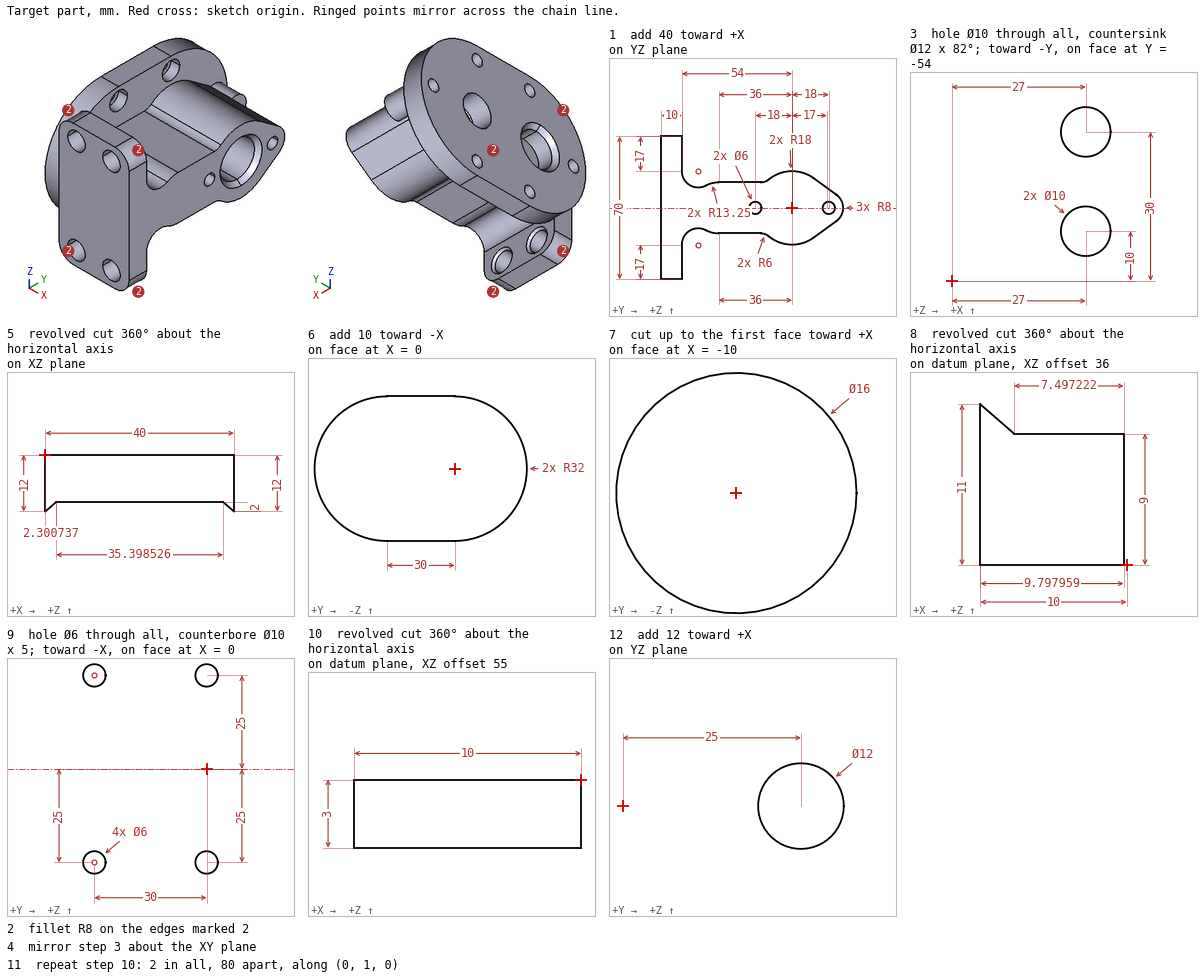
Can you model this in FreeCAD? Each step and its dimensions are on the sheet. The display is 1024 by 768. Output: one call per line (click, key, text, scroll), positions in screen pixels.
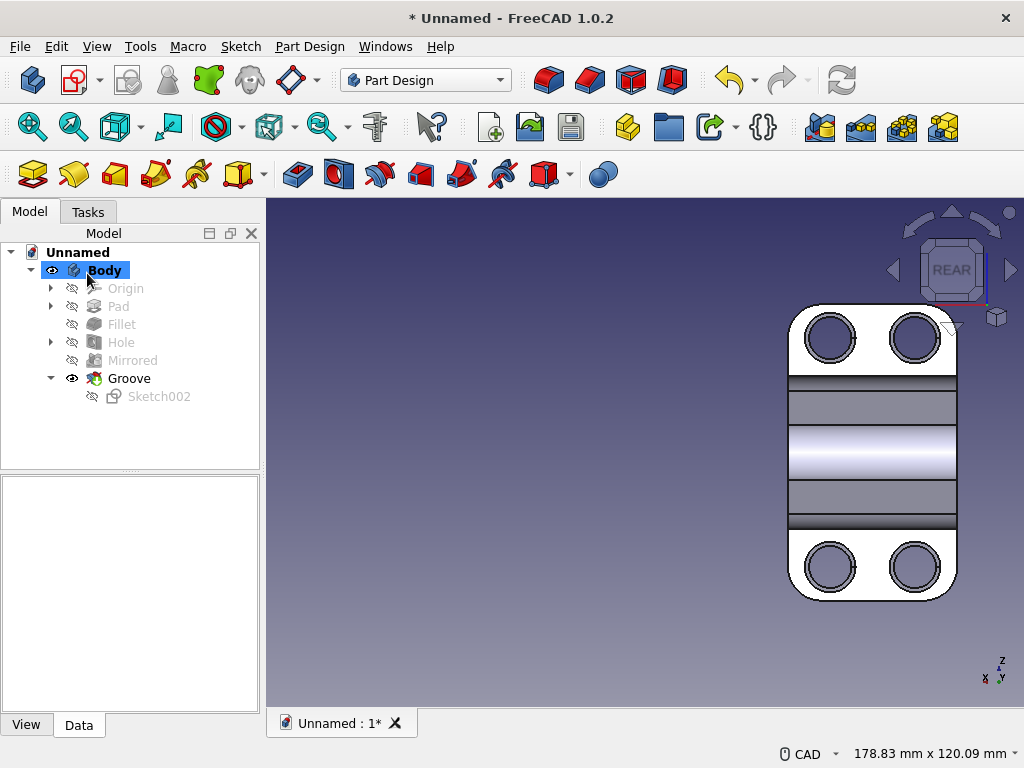
key(6)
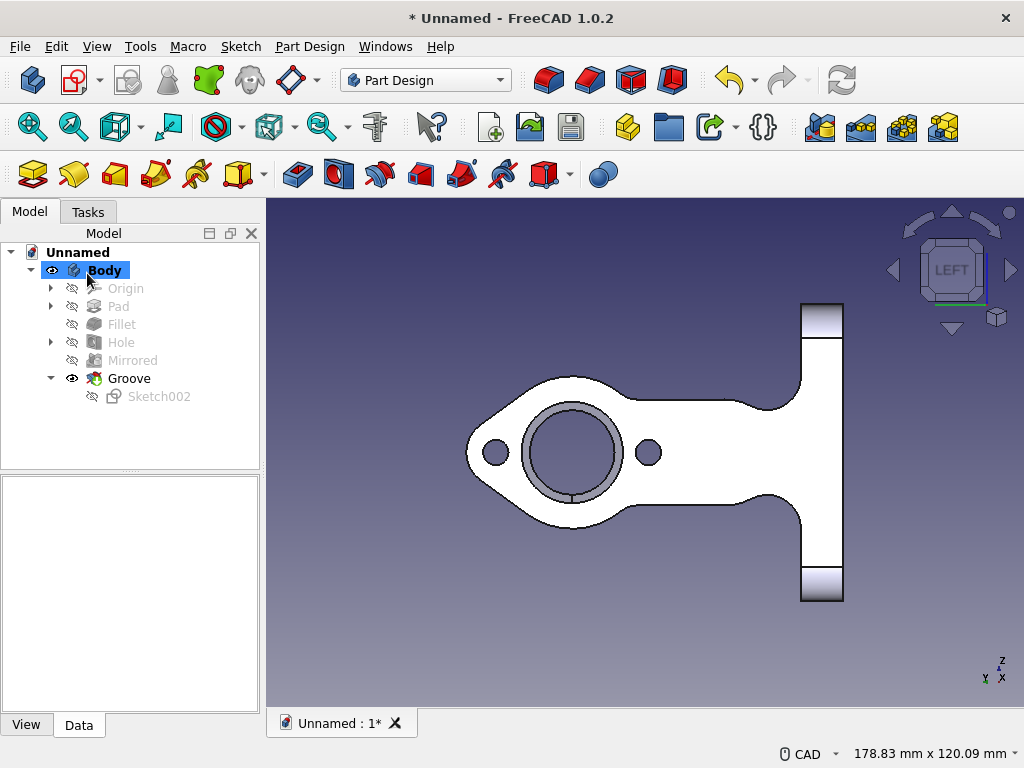
click(709, 451)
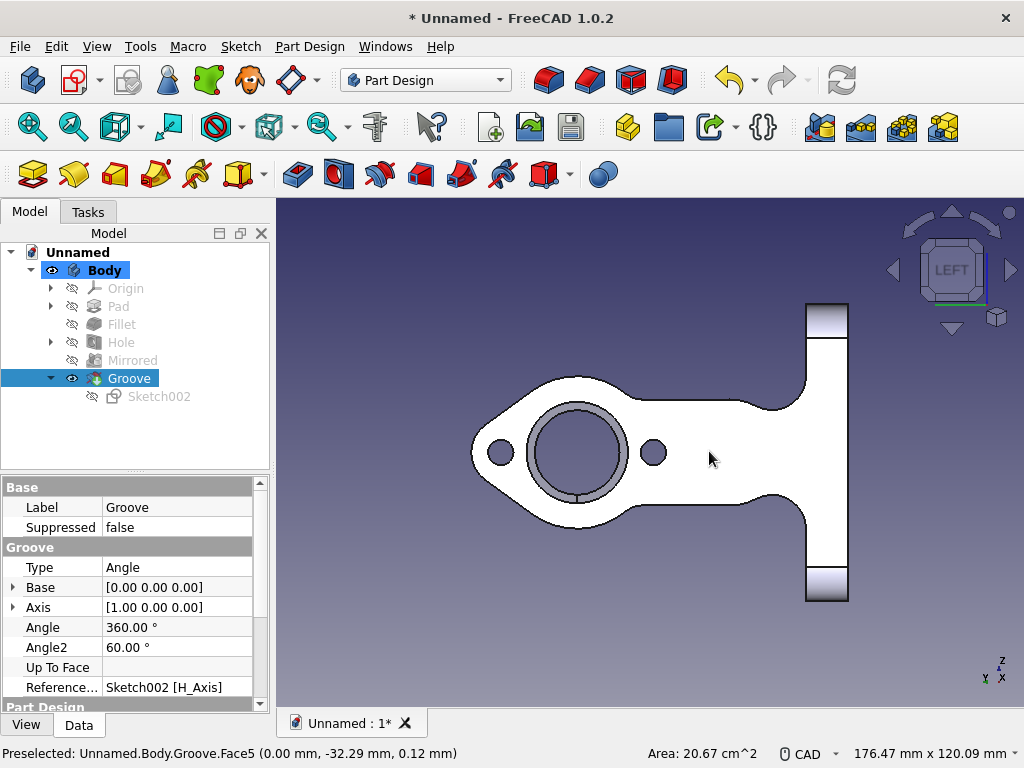
click(74, 80)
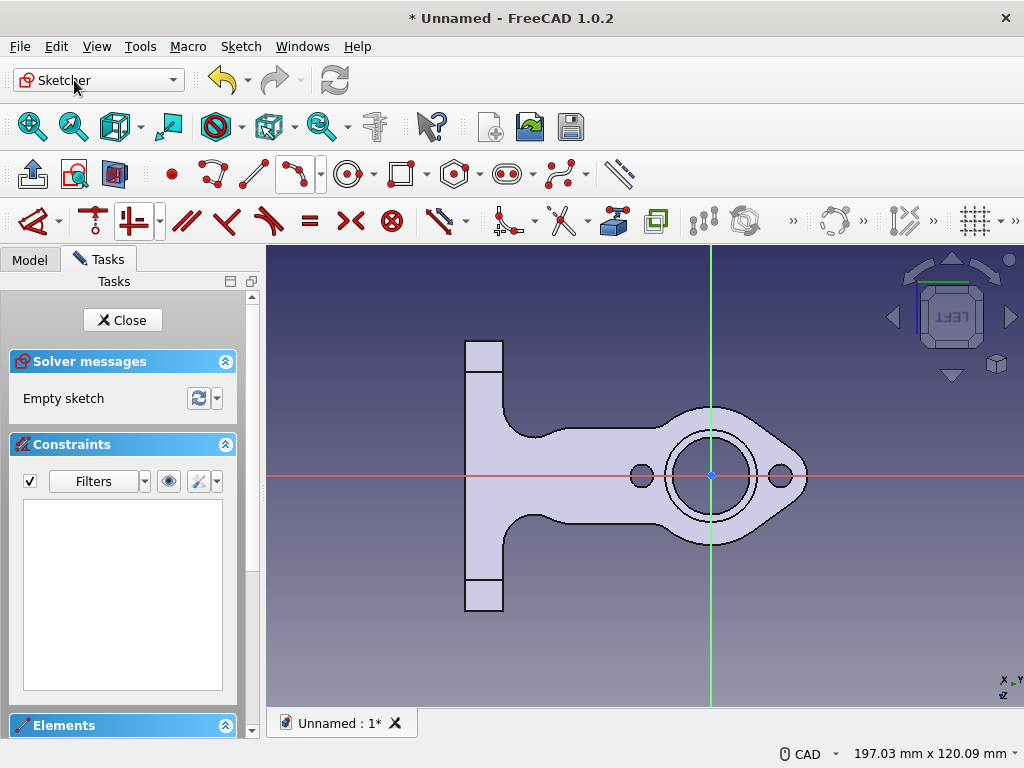
scroll(294, 476, down, 1)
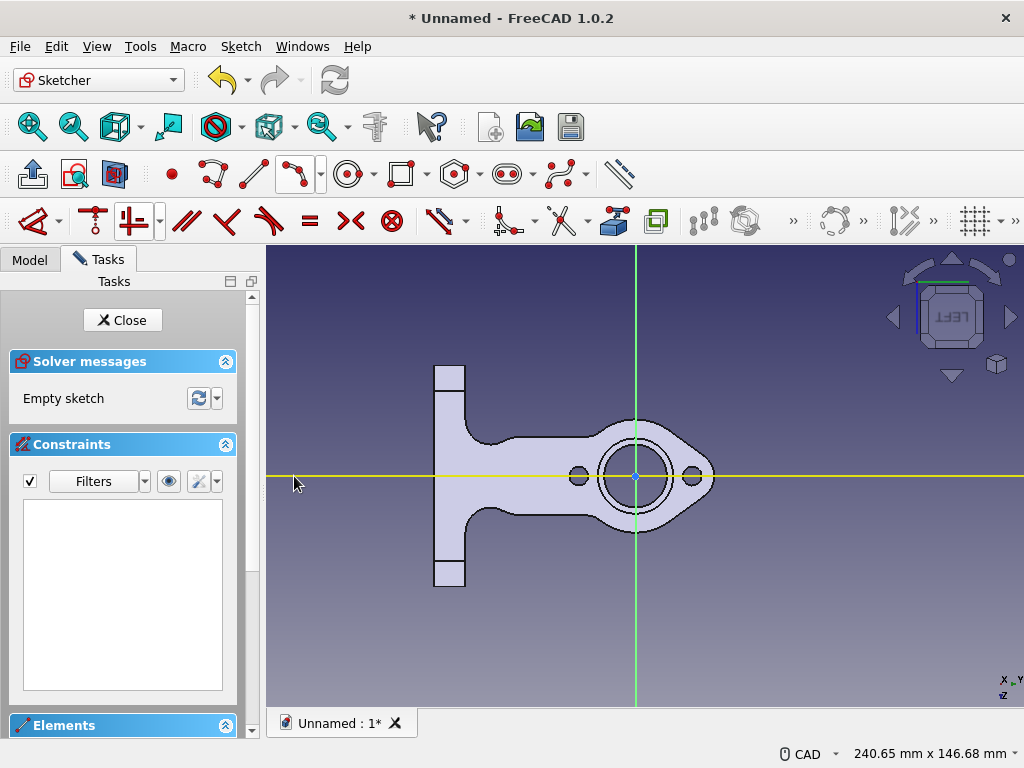
click(506, 174)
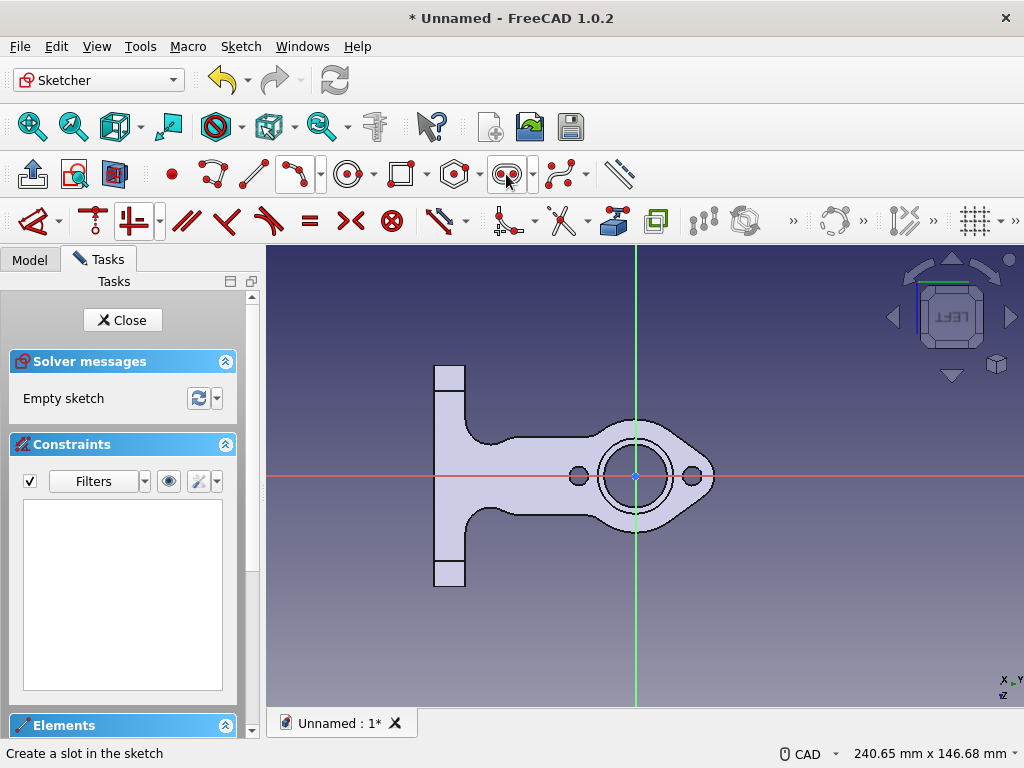
click(636, 476)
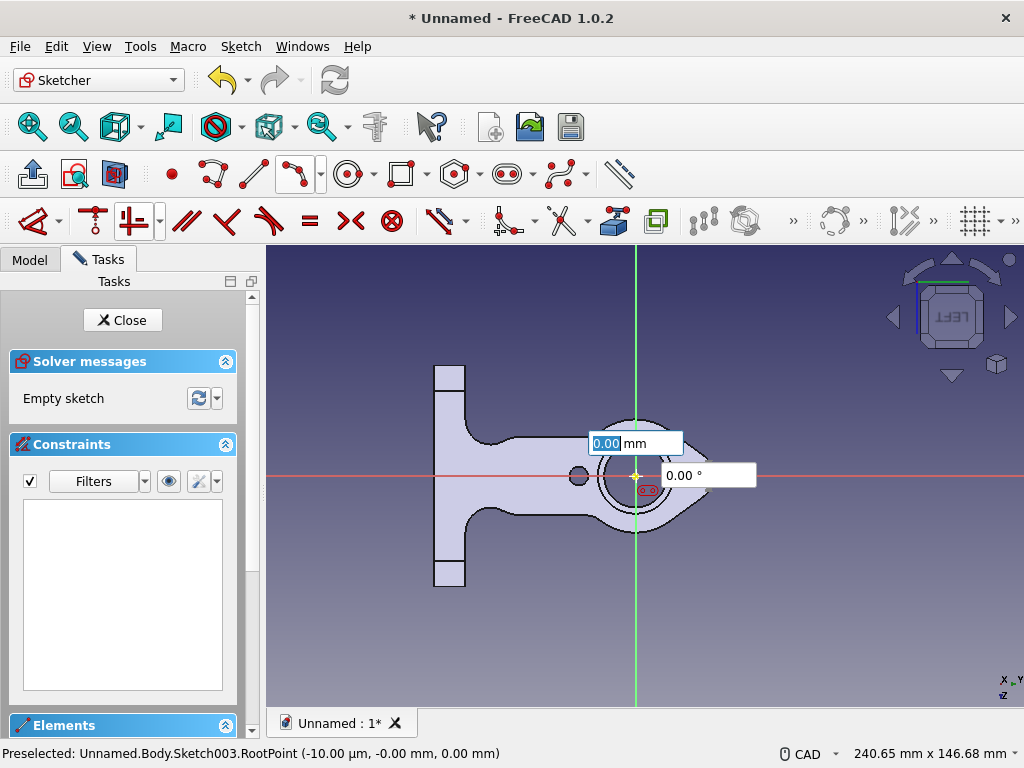
click(541, 467)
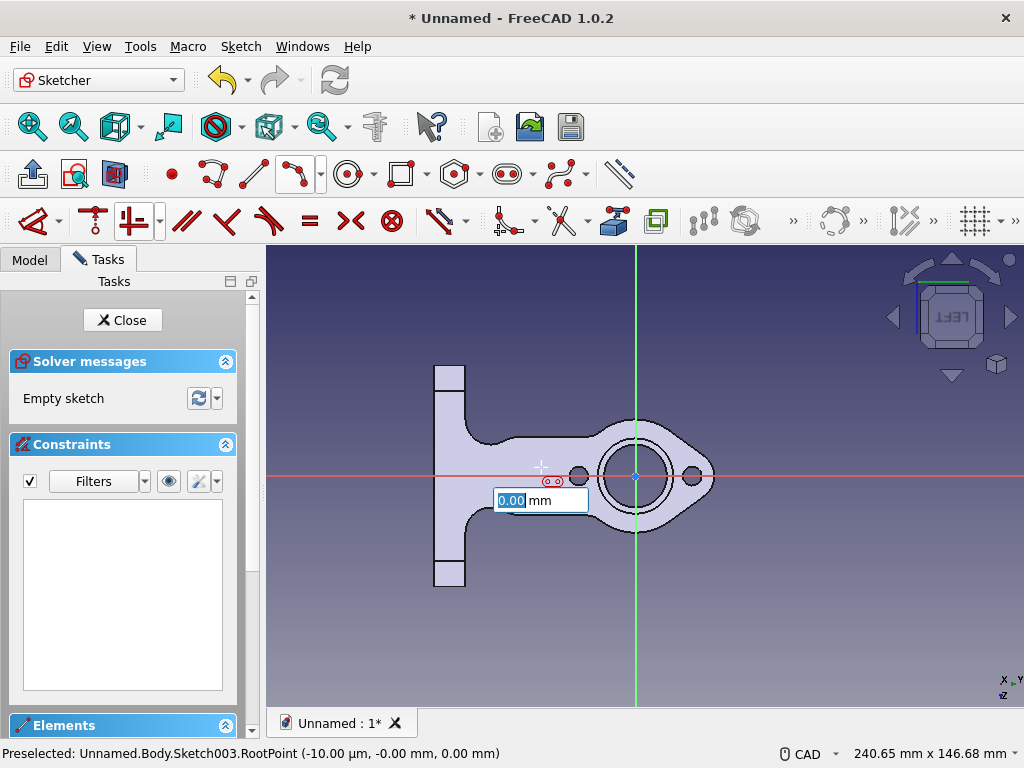
click(588, 577)
key(Escape)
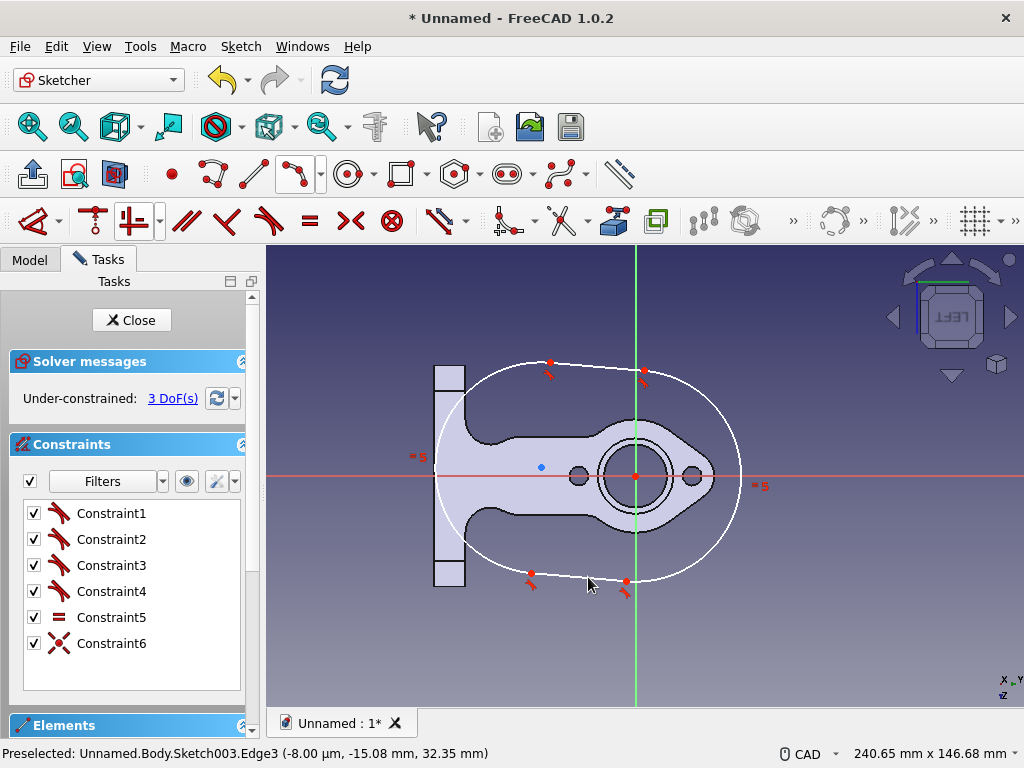
click(598, 579)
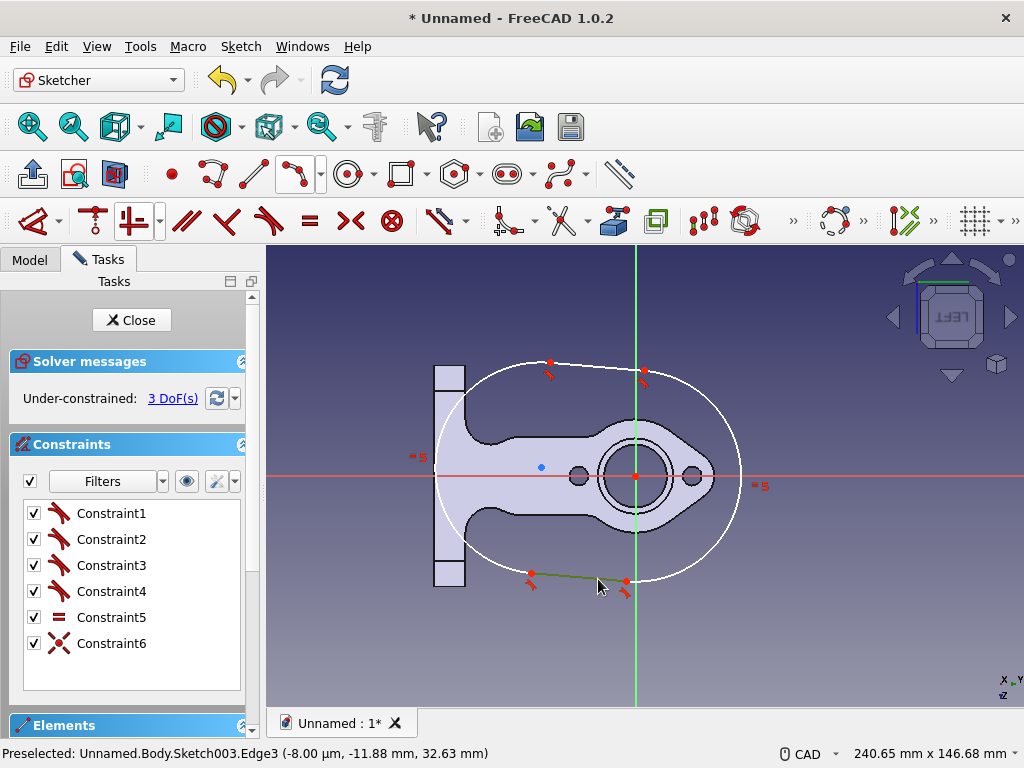
click(160, 222)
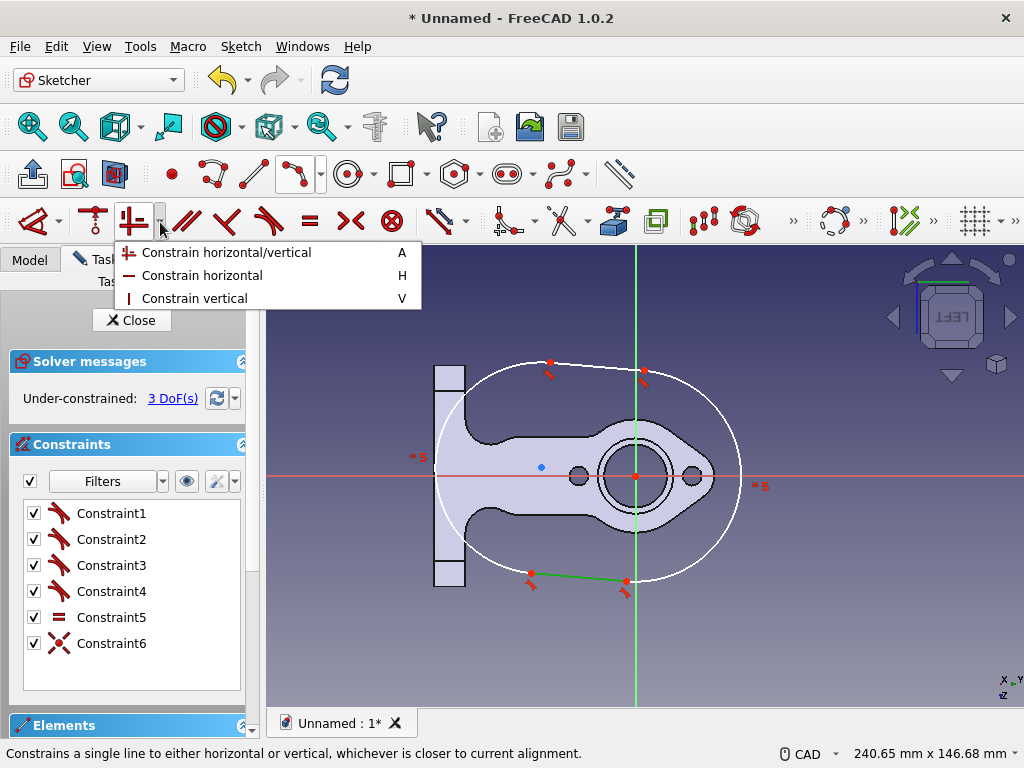
click(268, 276)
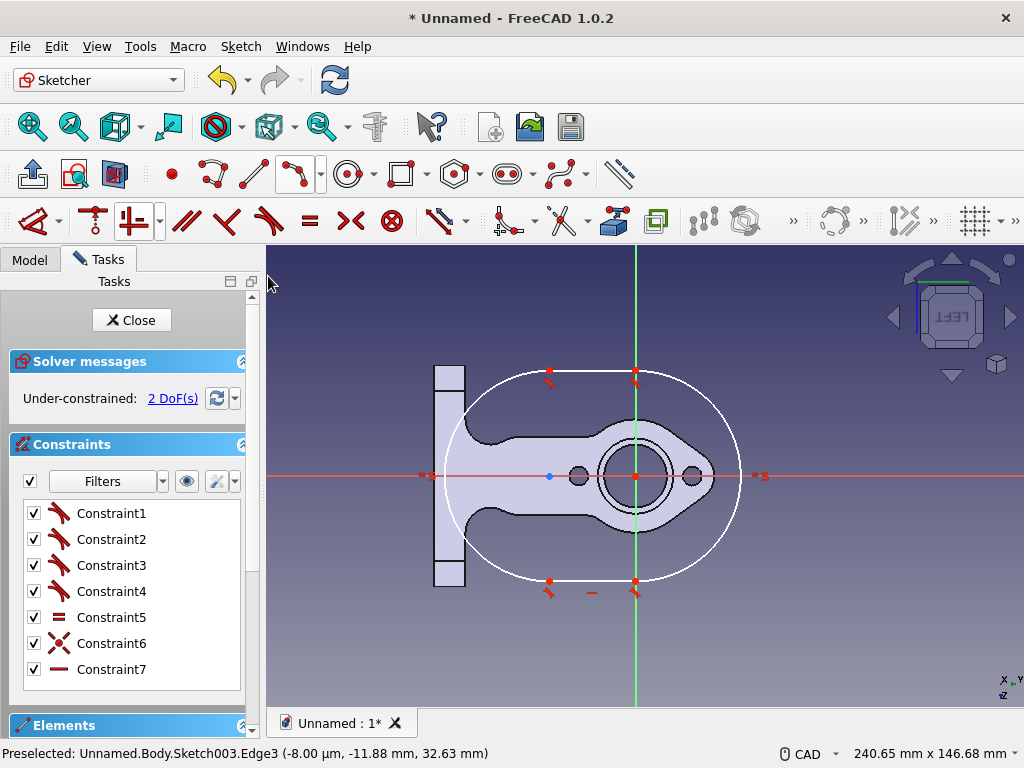
click(32, 222)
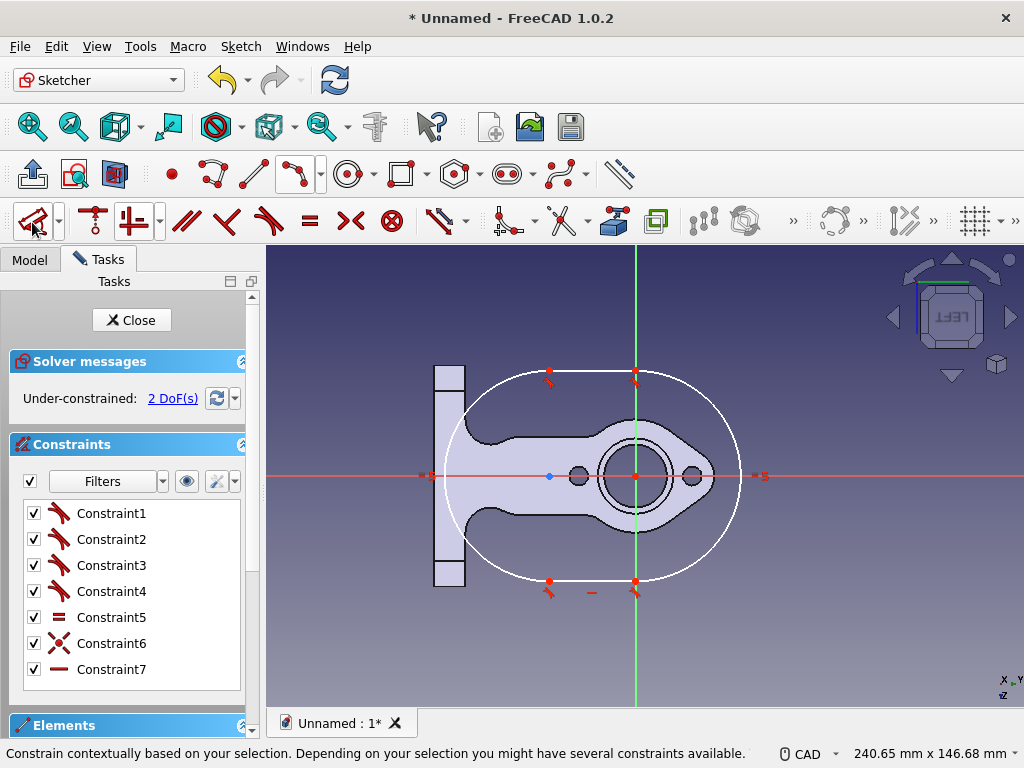
click(721, 538)
click(747, 557)